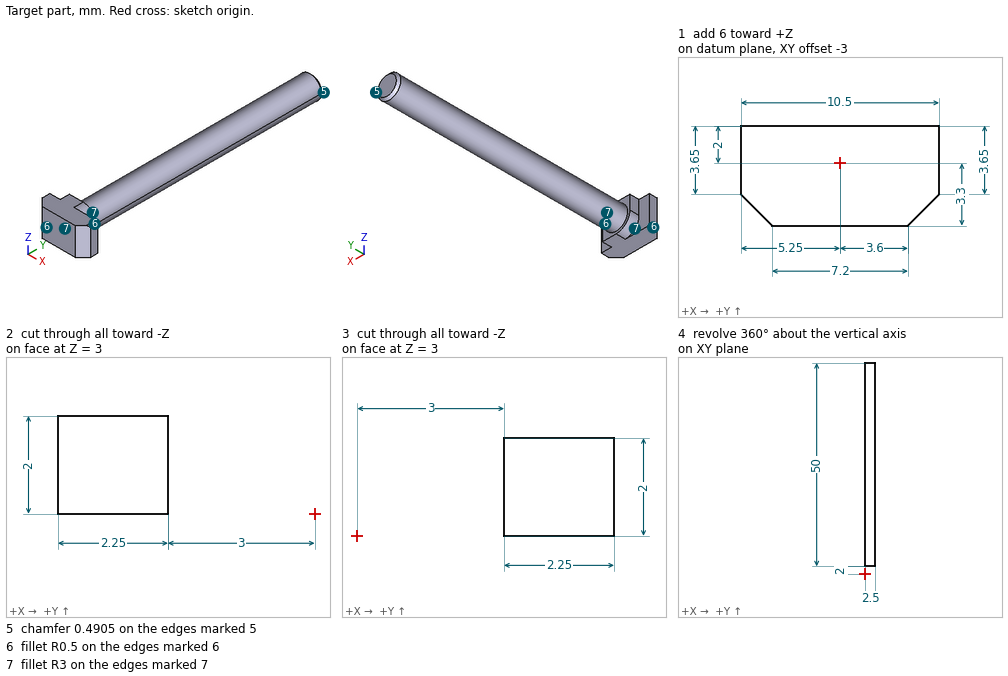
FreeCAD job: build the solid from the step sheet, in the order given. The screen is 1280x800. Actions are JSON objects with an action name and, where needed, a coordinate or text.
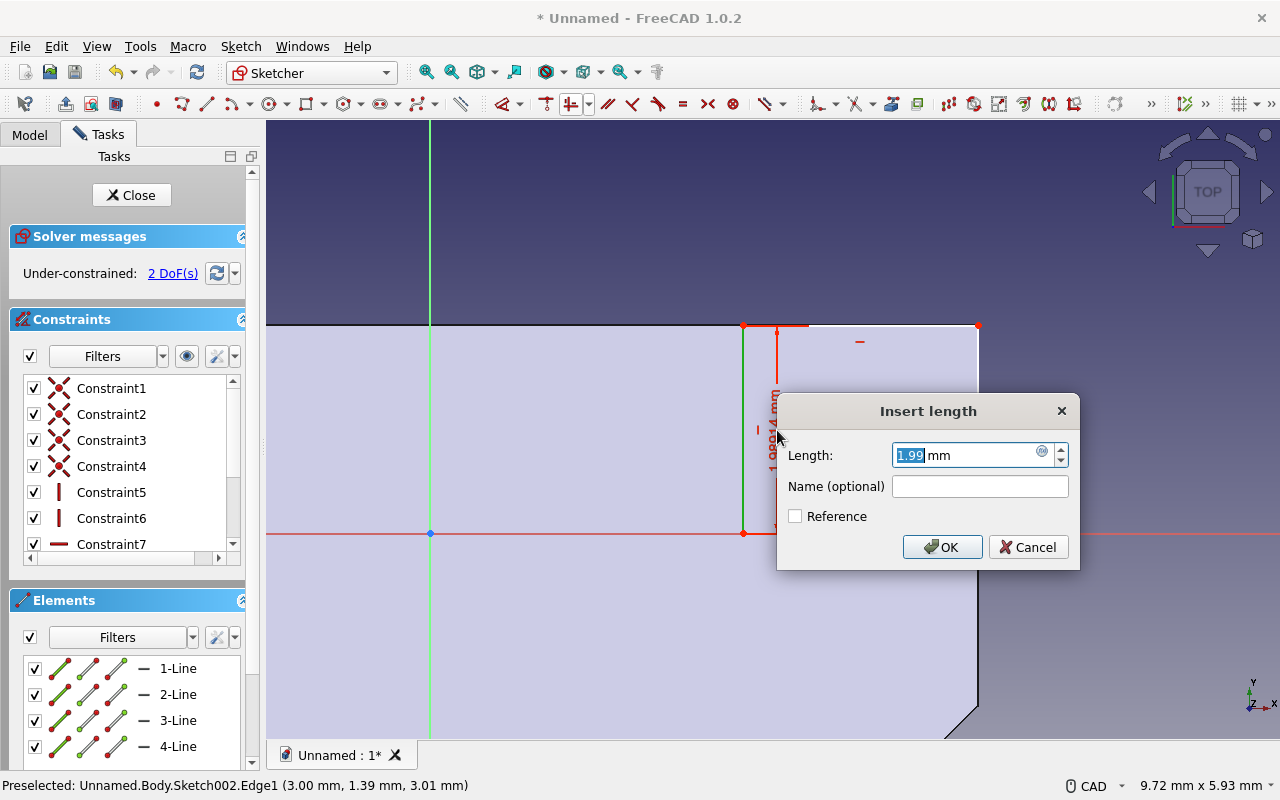
{"action": "type", "text": "2"}
{"action": "key", "text": "Return"}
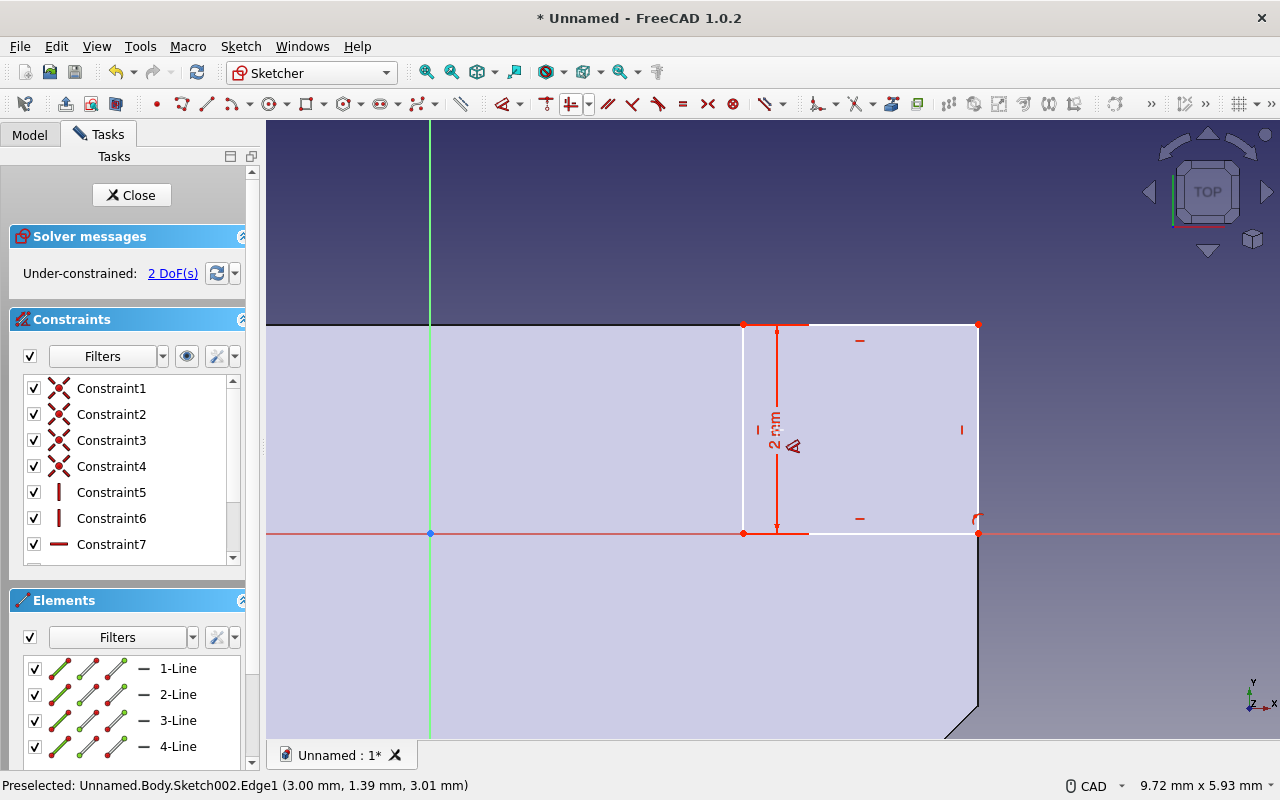
{"action": "left_click", "coordinate": [743, 325]}
{"action": "left_click", "coordinate": [587, 568]}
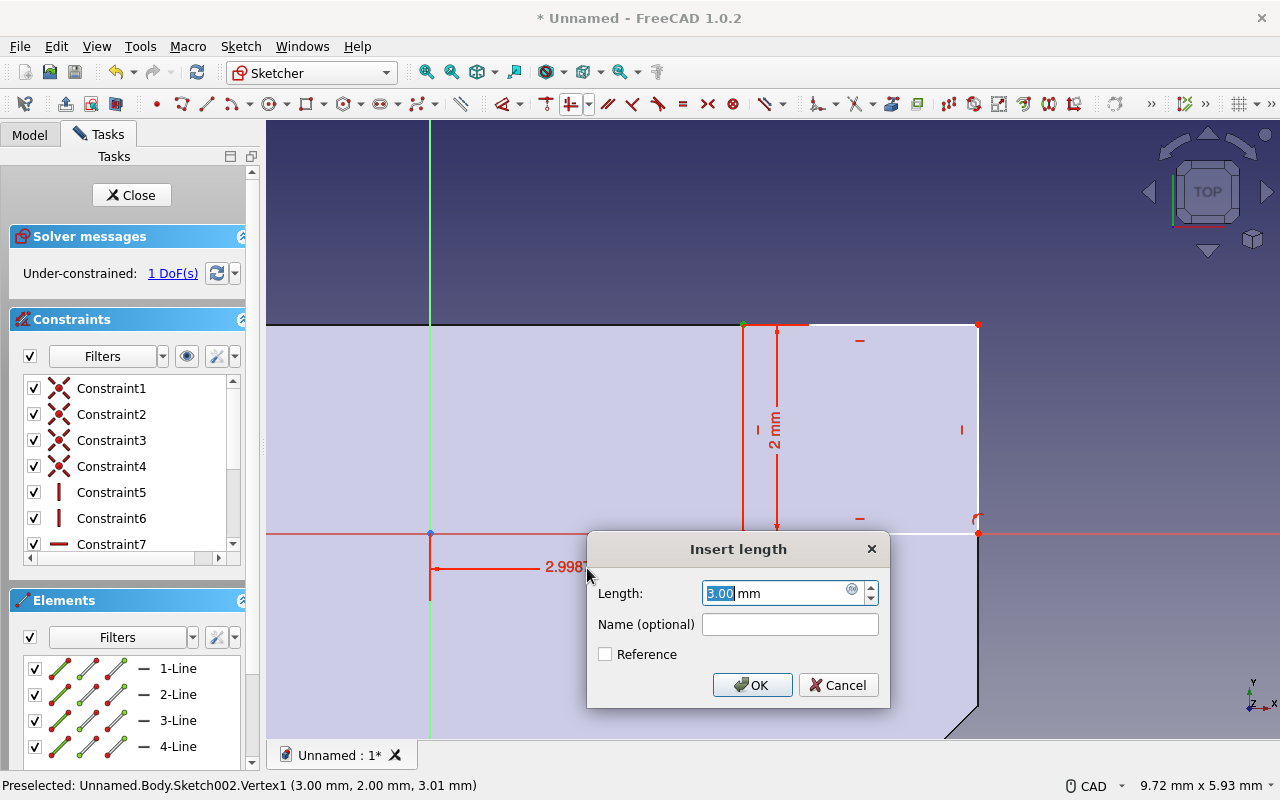
{"action": "type", "text": "3"}
{"action": "key", "text": "Return"}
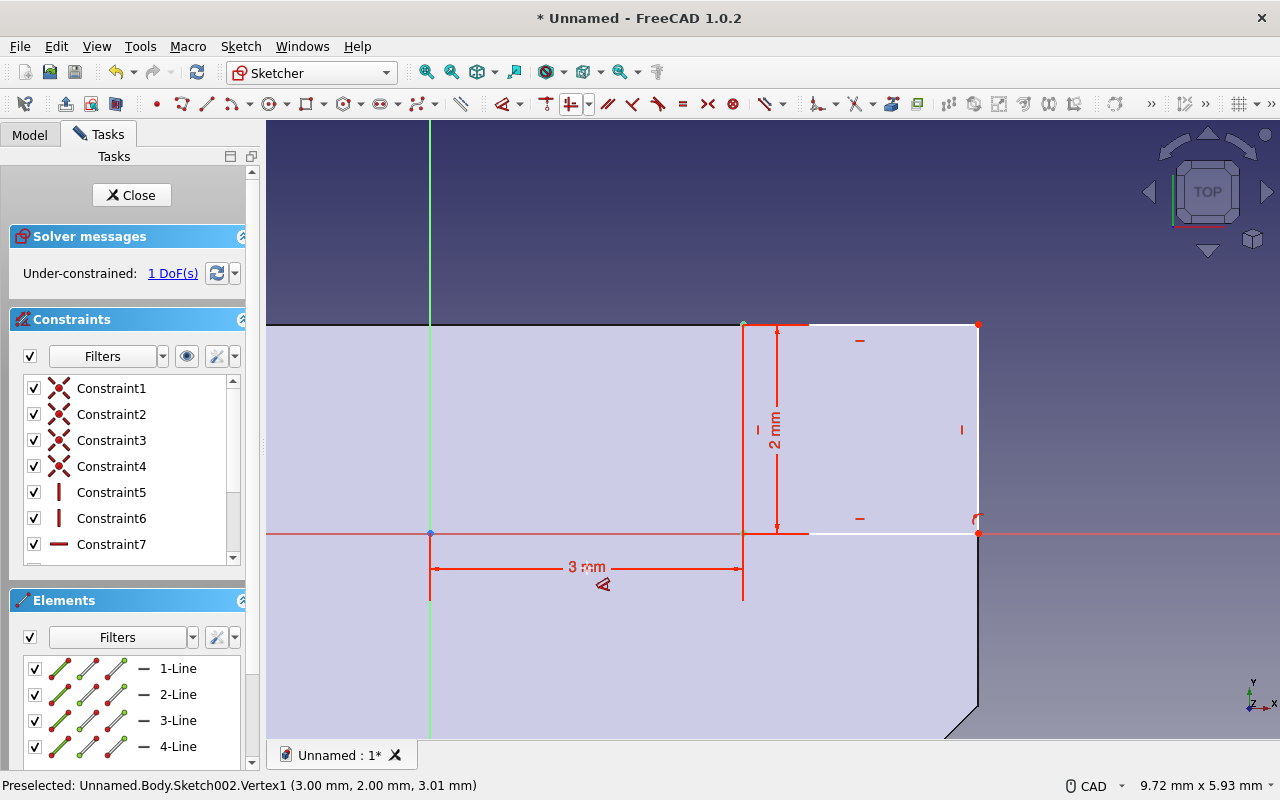
{"action": "left_click", "coordinate": [814, 534]}
{"action": "left_click", "coordinate": [861, 568]}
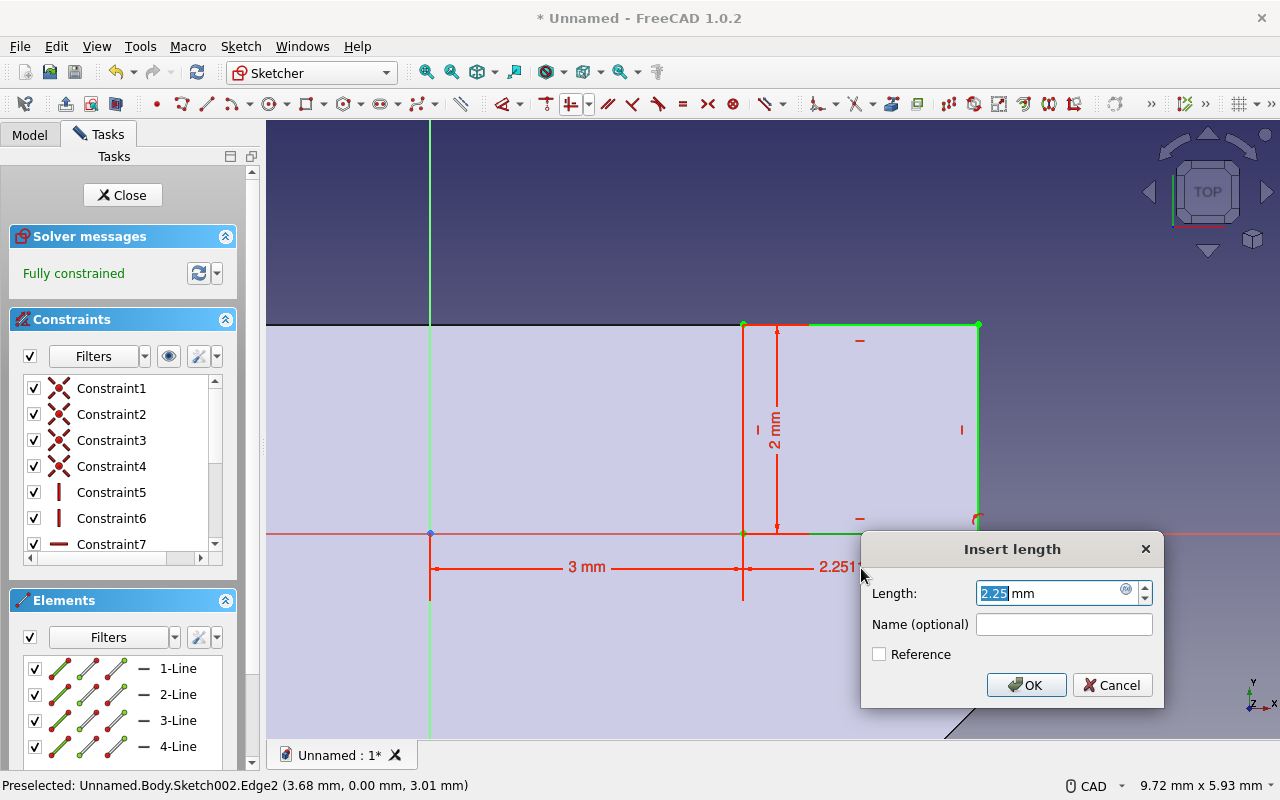
{"action": "type", "text": "2.25"}
{"action": "key", "text": "Return"}
{"action": "key", "text": "Escape"}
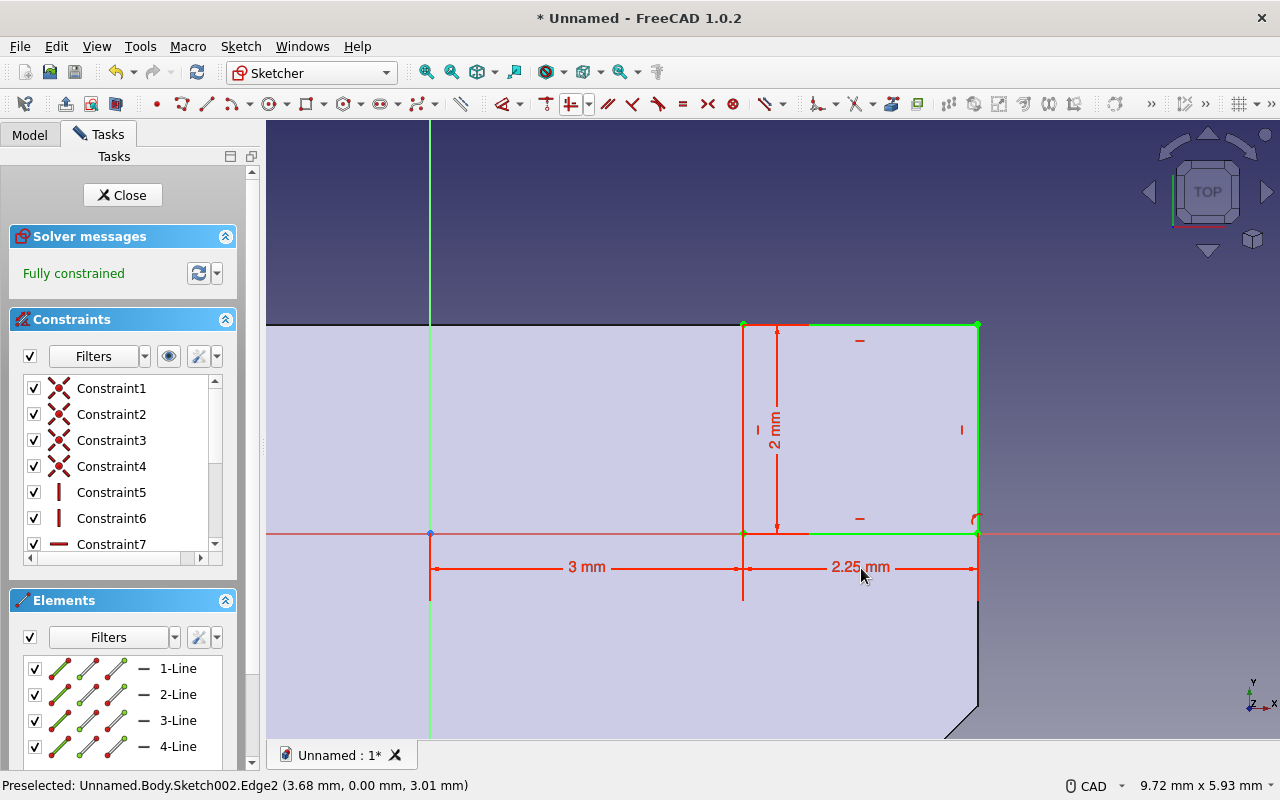
{"action": "left_click", "coordinate": [123, 195]}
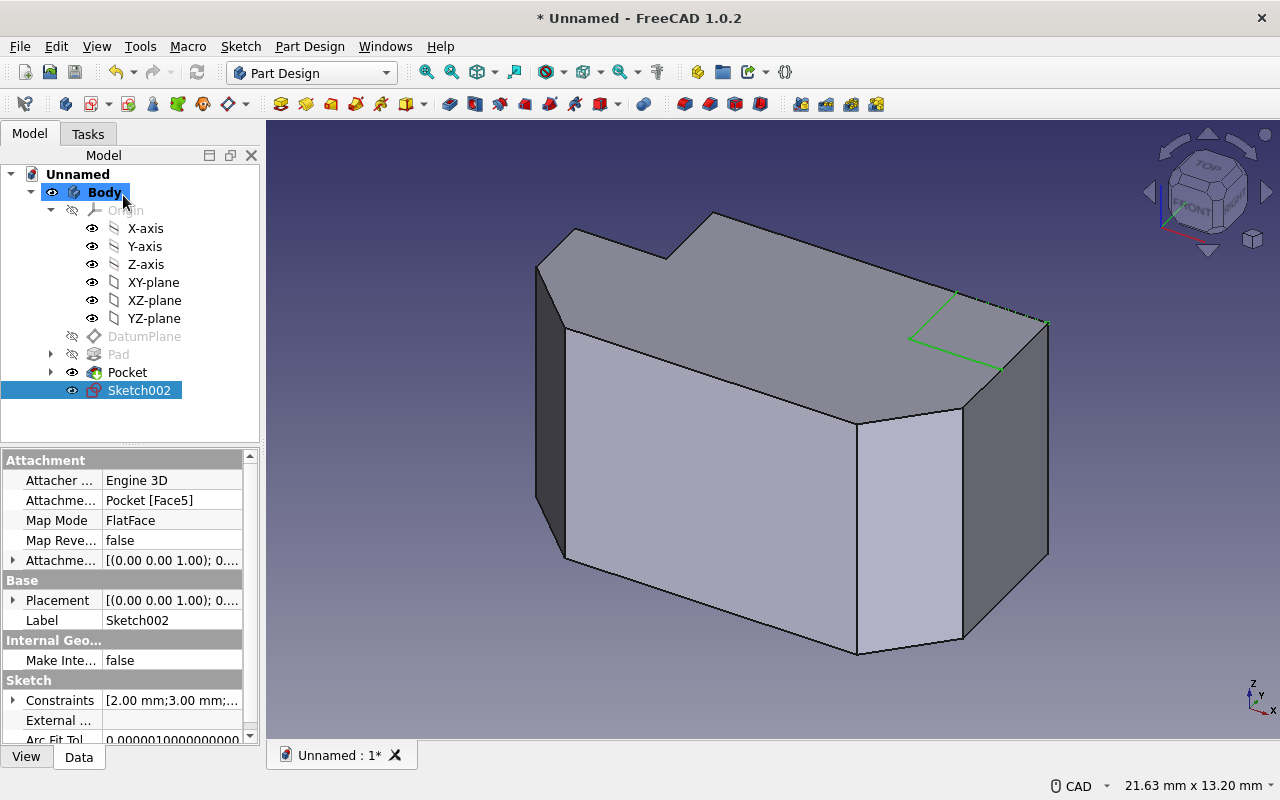
{"action": "left_click", "coordinate": [450, 104]}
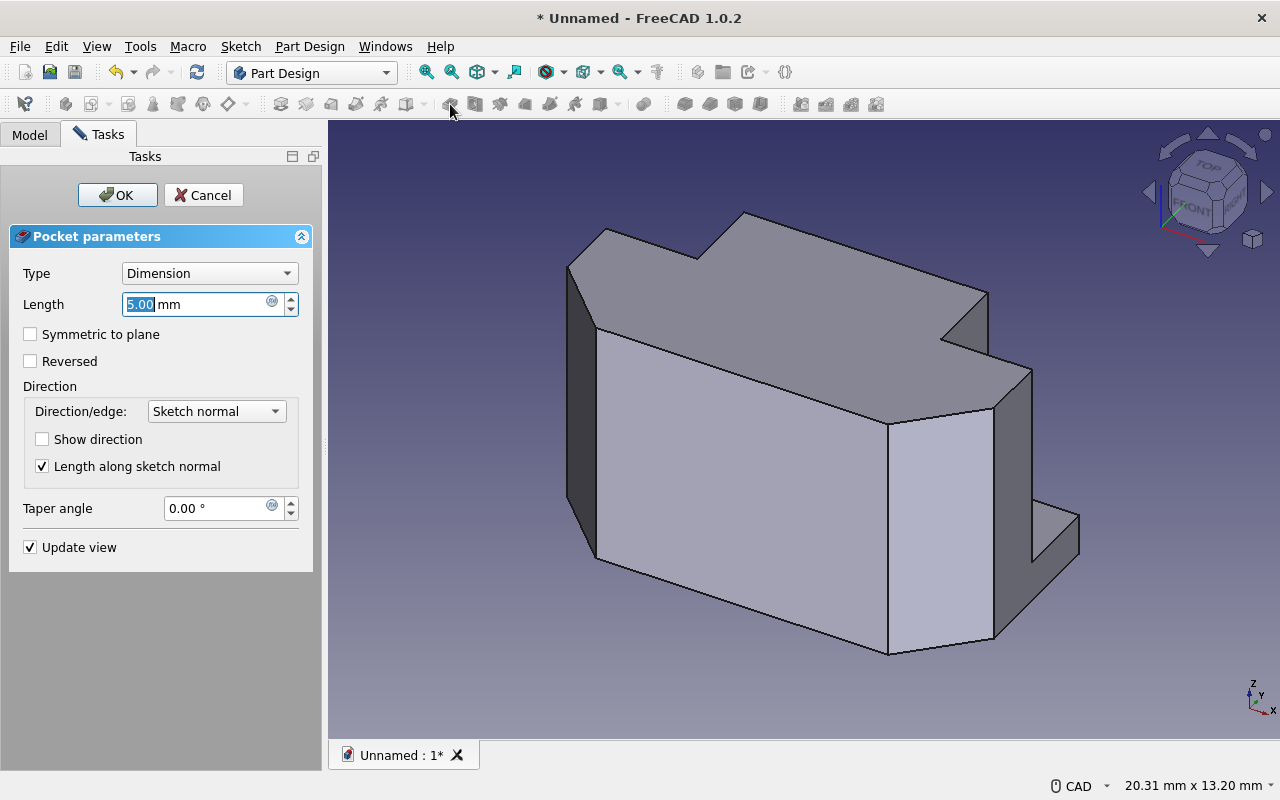
{"action": "left_click", "coordinate": [210, 274]}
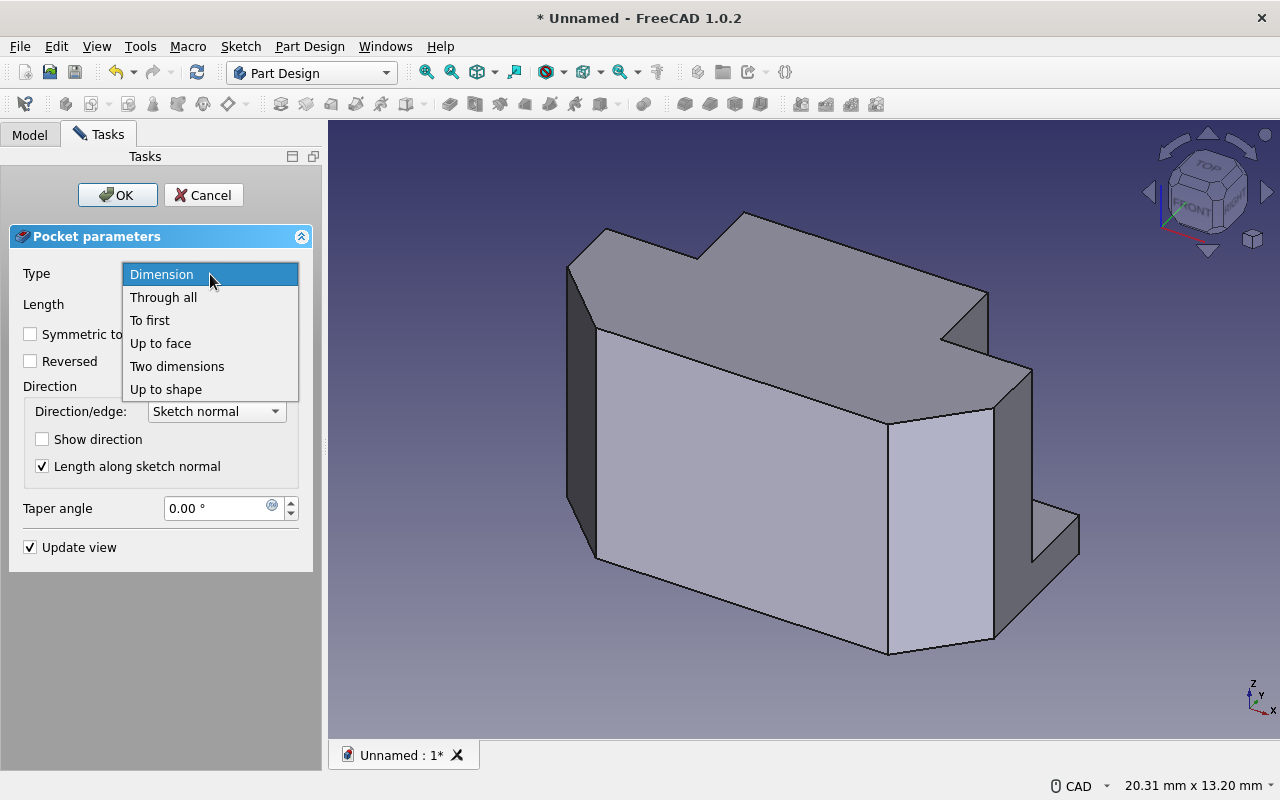
{"action": "left_click", "coordinate": [208, 298]}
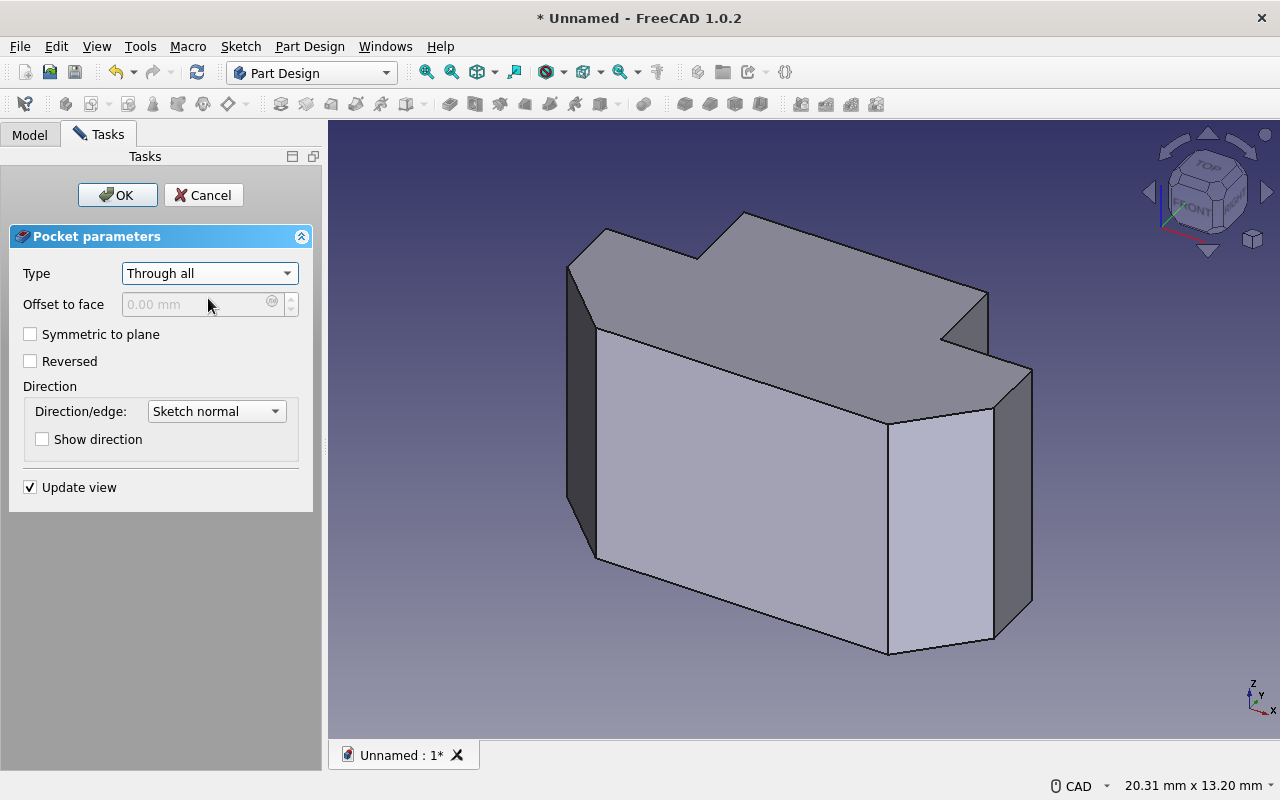
{"action": "left_click", "coordinate": [118, 195]}